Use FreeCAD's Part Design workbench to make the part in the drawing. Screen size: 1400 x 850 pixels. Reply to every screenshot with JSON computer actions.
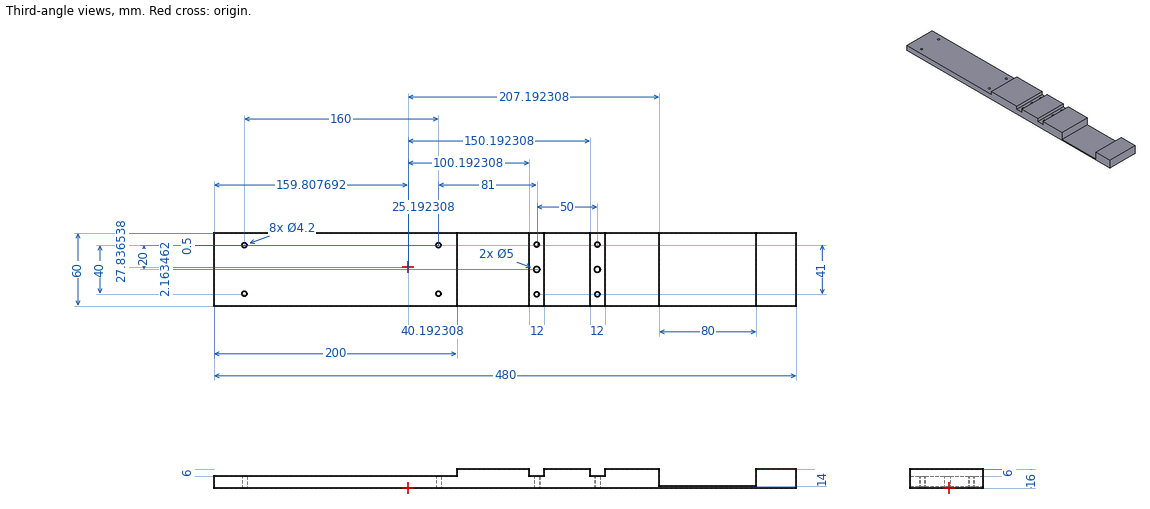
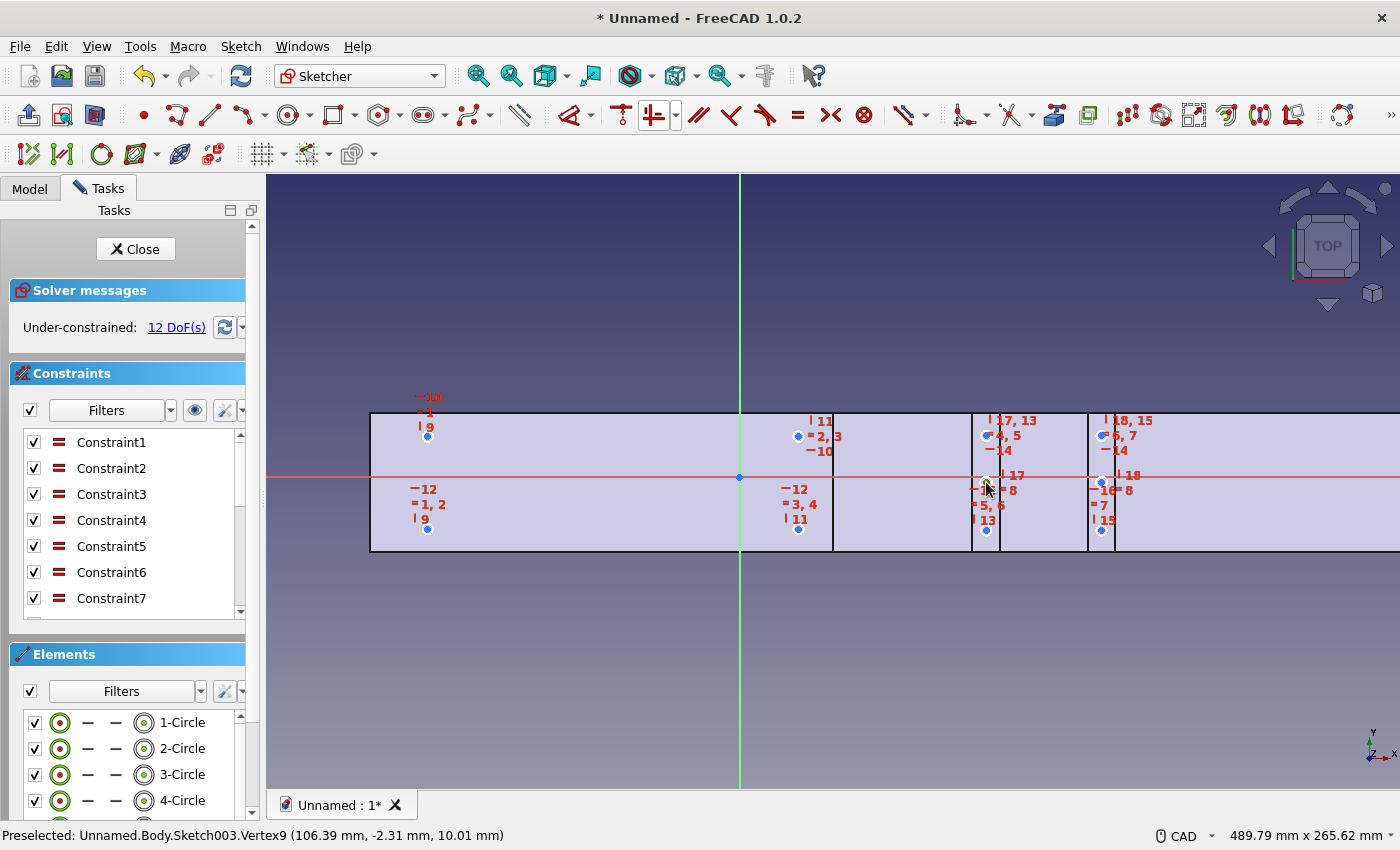
{"action": "left_click", "coordinate": [1102, 482]}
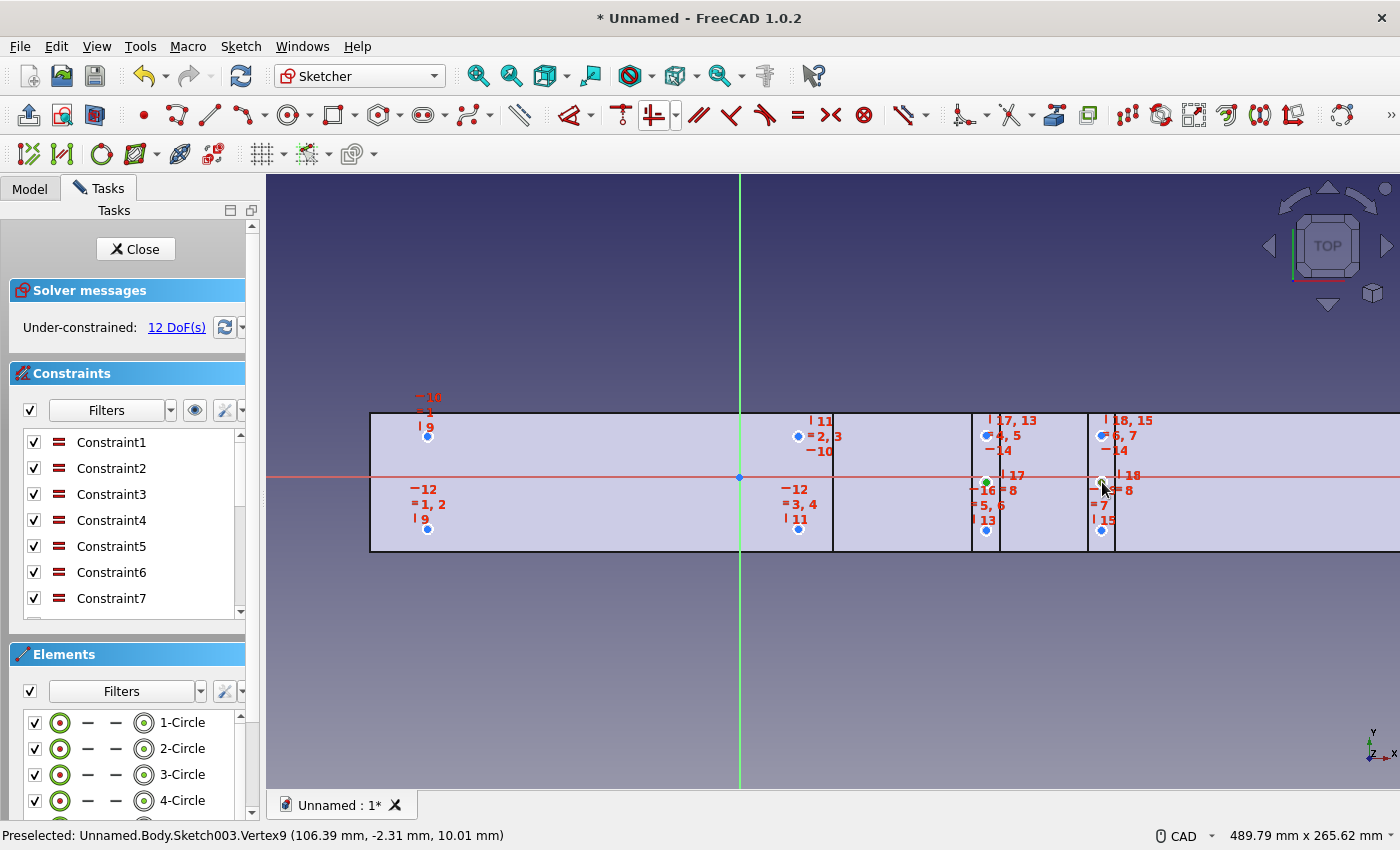
{"action": "key", "text": "h"}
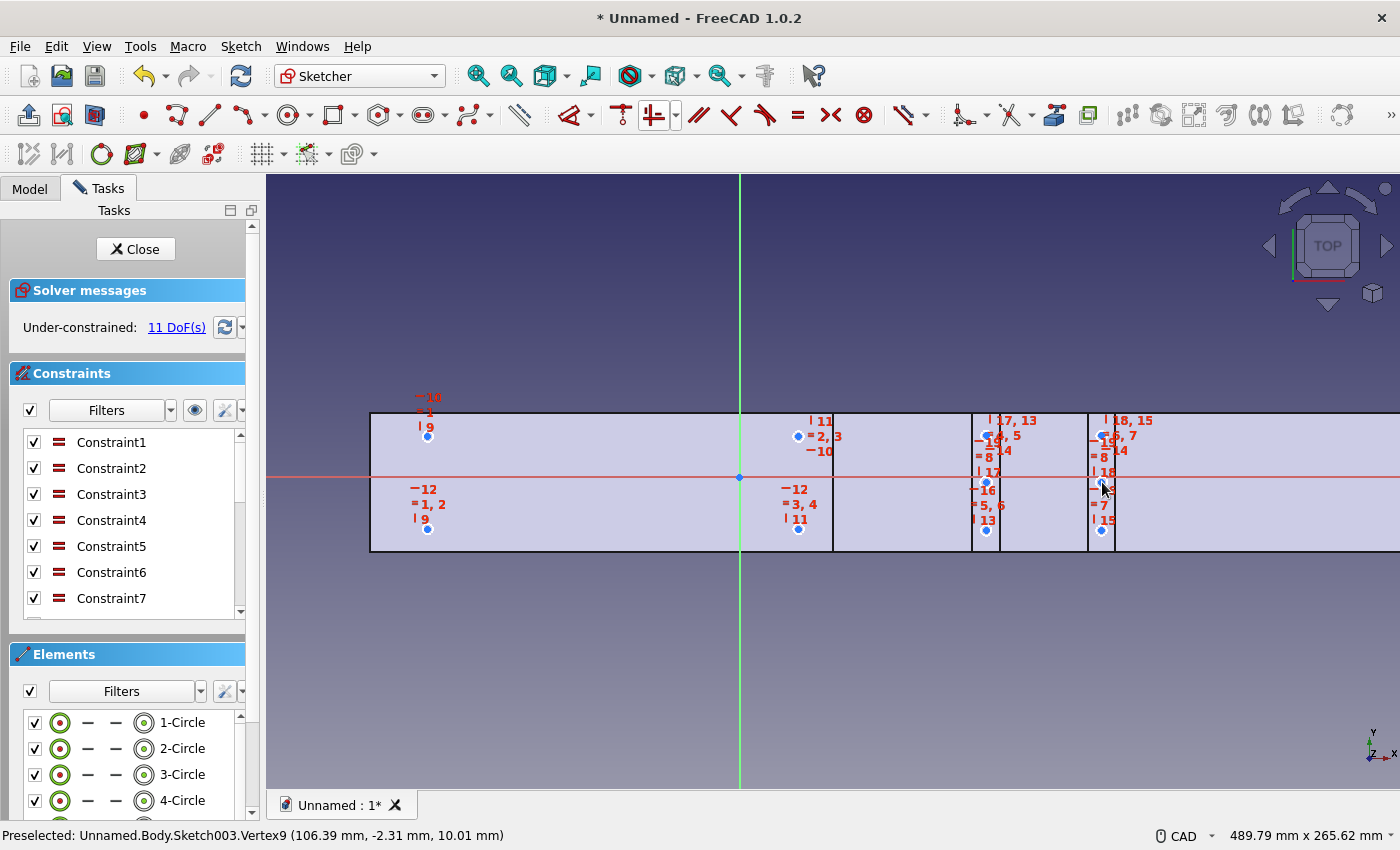
{"action": "key", "text": "d"}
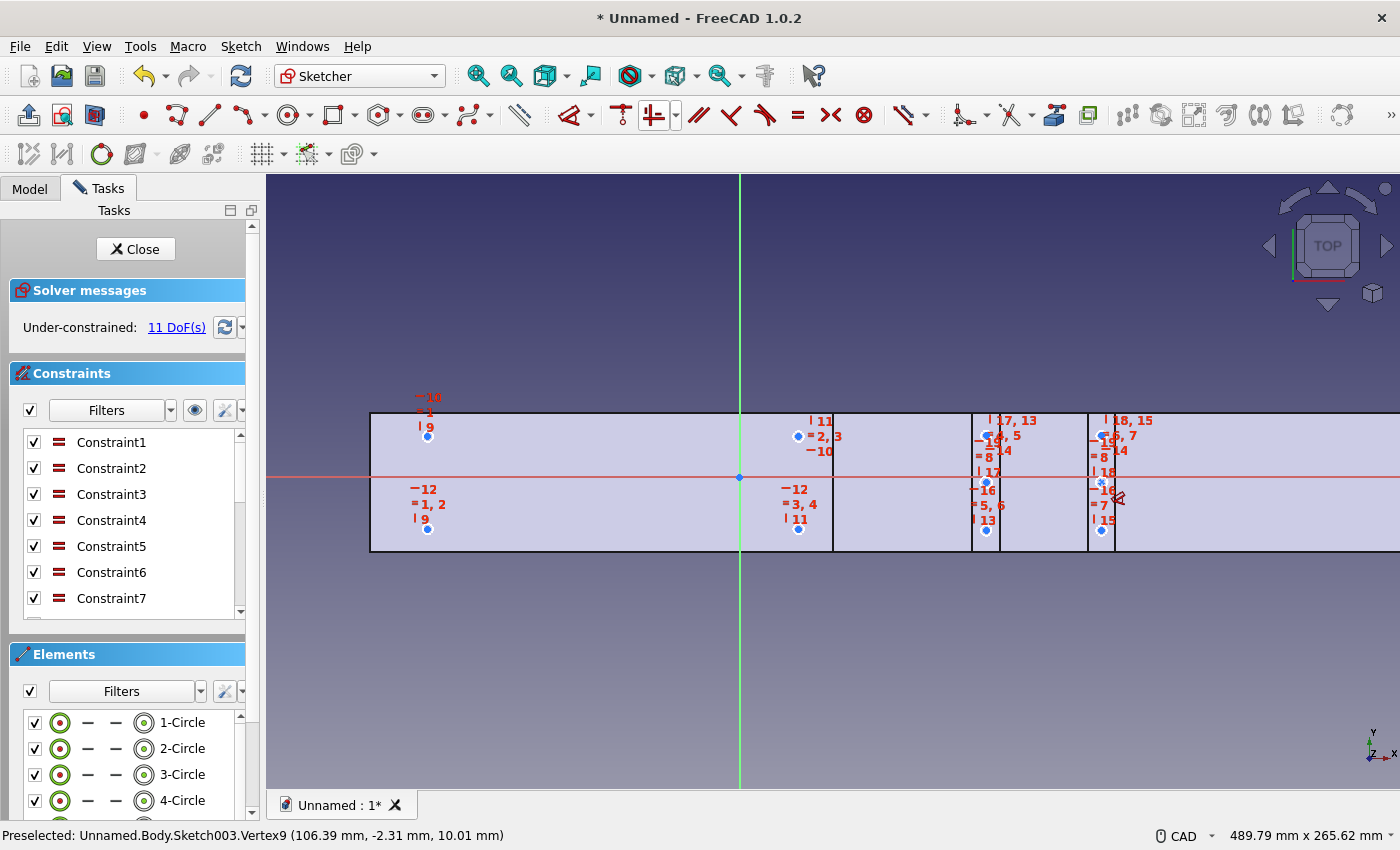
{"action": "scroll", "coordinate": [423, 436], "scroll_direction": "up", "scroll_amount": 8}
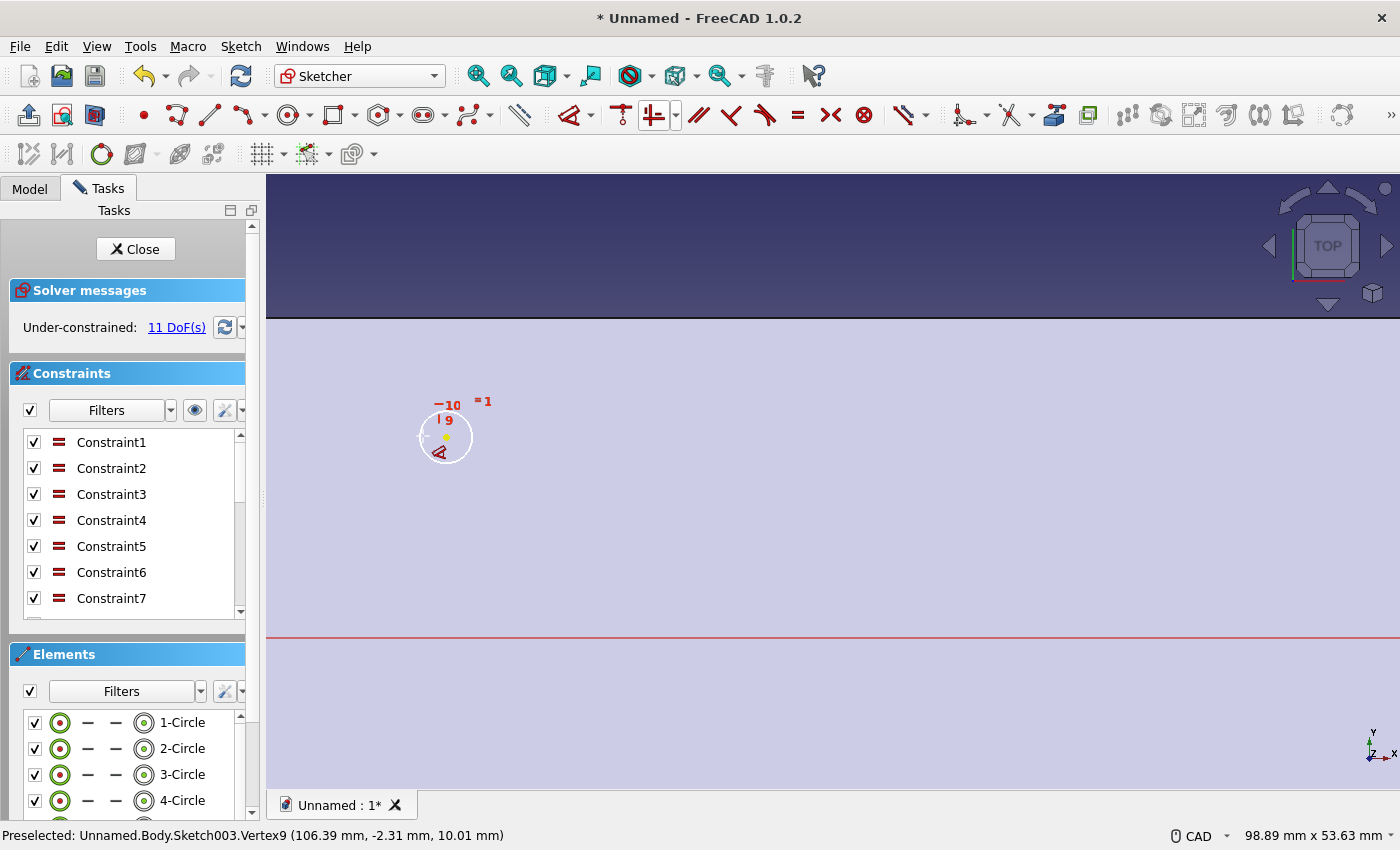
{"action": "left_click", "coordinate": [420, 437]}
{"action": "left_click", "coordinate": [388, 437]}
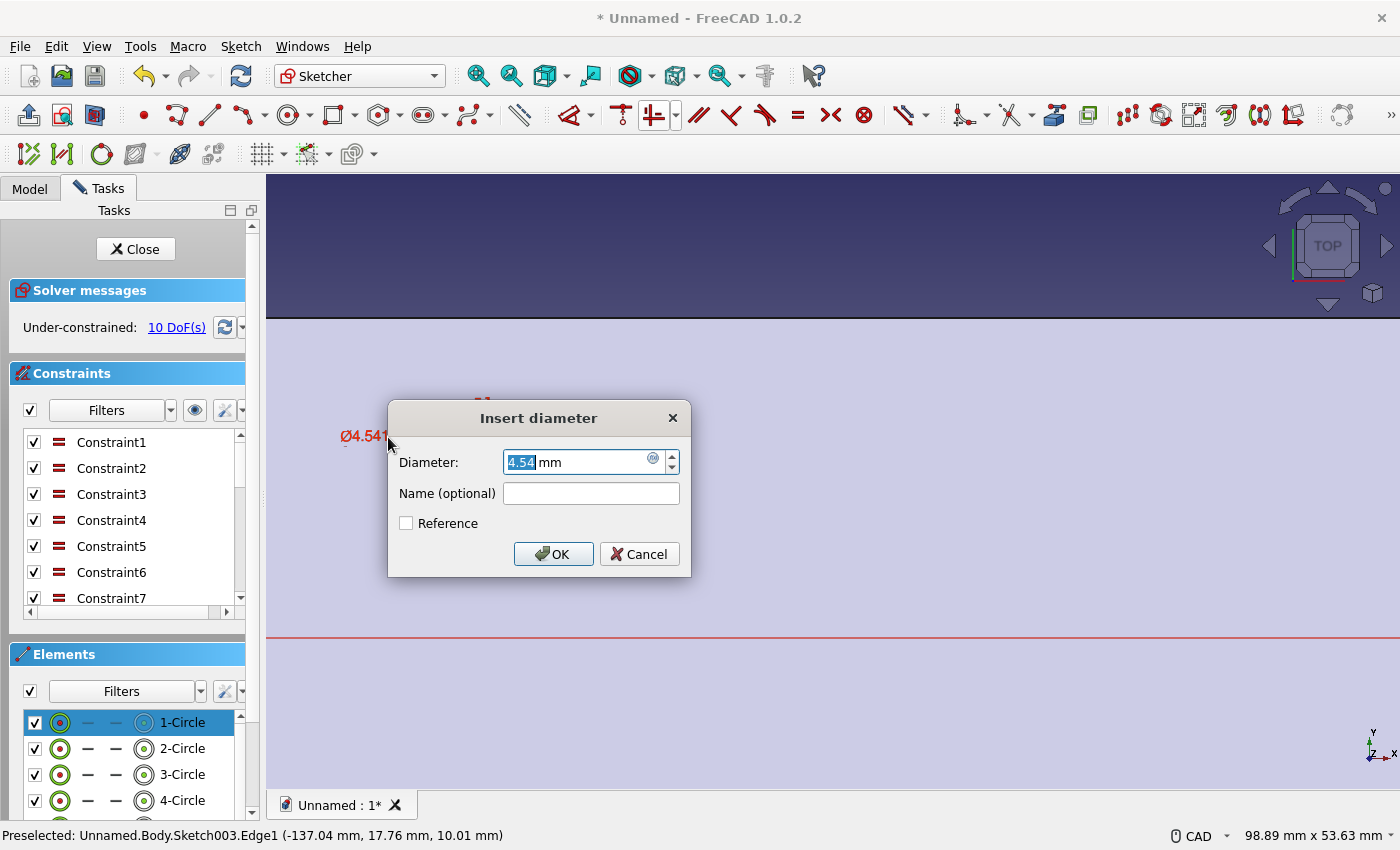
{"action": "type", "text": "4.2"}
{"action": "key", "text": "Return"}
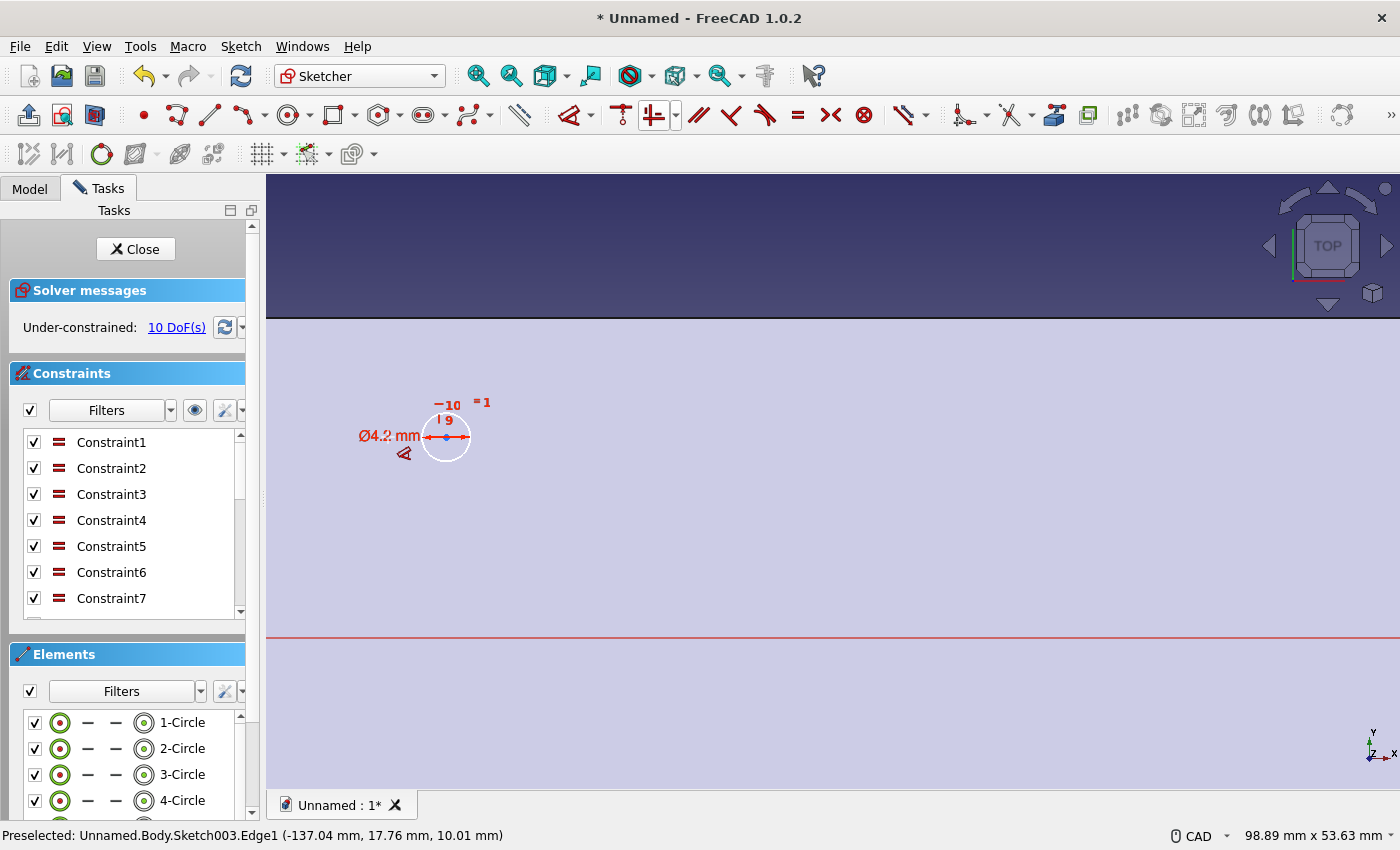
{"action": "scroll", "coordinate": [422, 436], "scroll_direction": "down", "scroll_amount": 8}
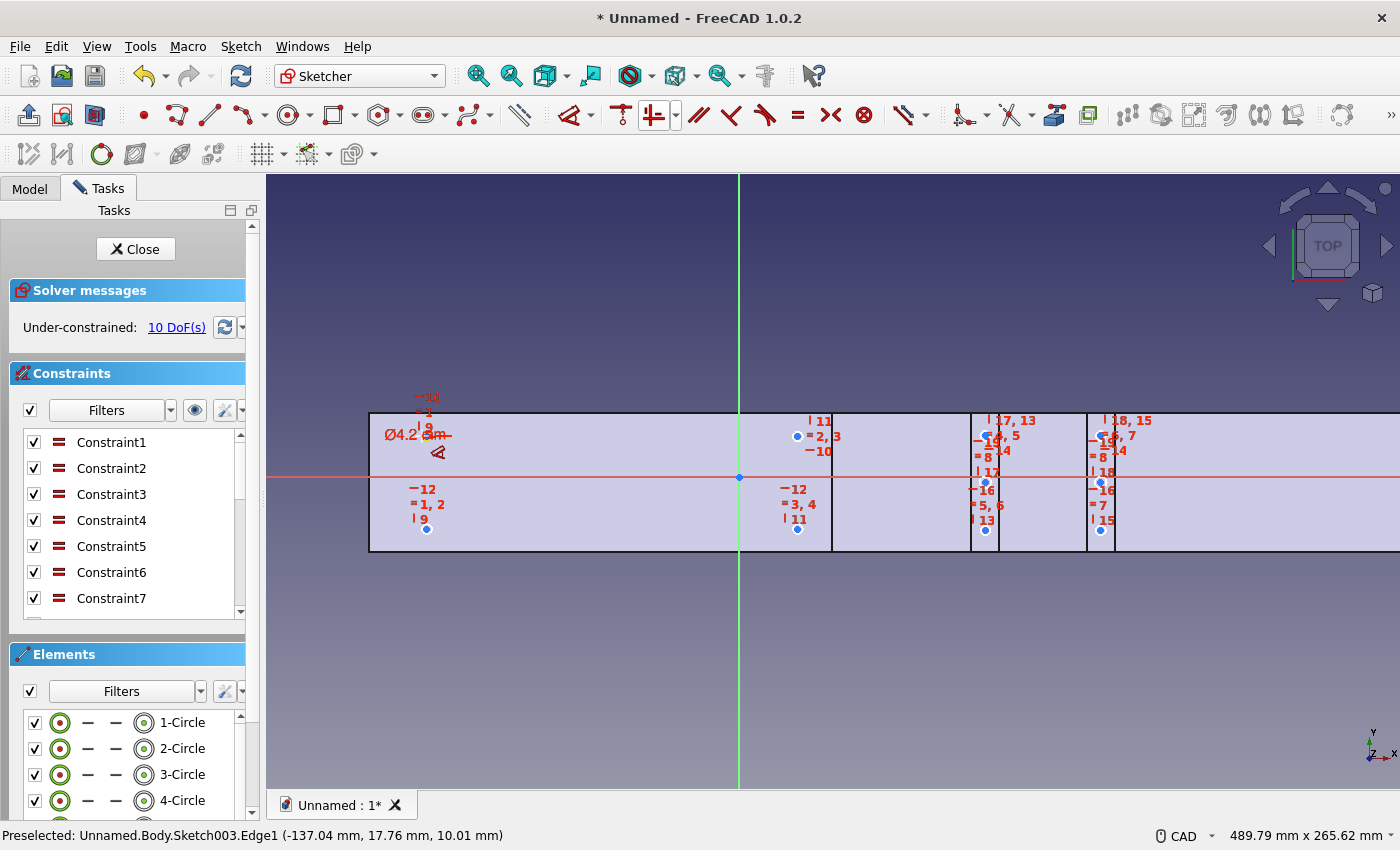
{"action": "scroll", "coordinate": [981, 487], "scroll_direction": "up", "scroll_amount": 7}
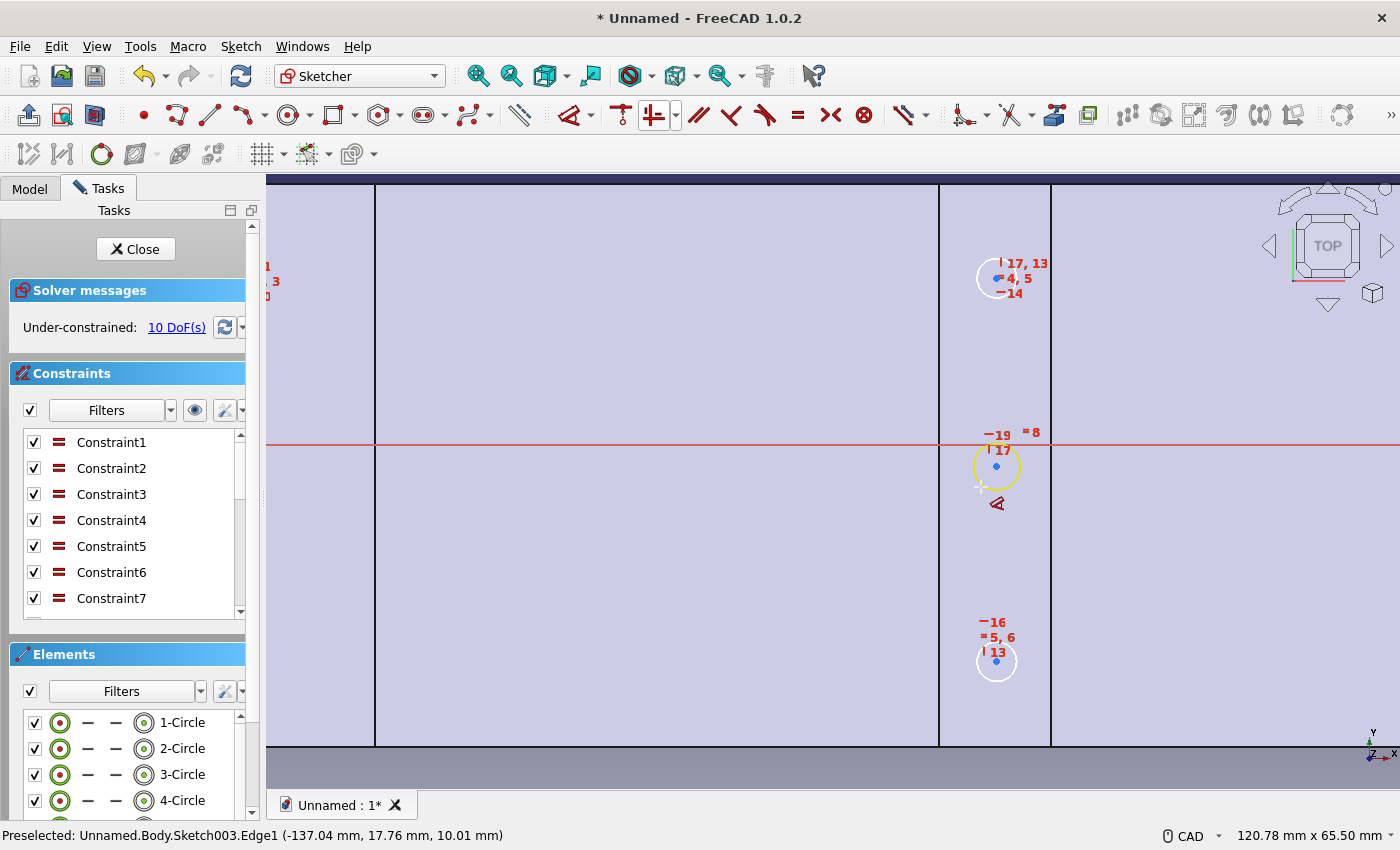
{"action": "left_click", "coordinate": [980, 483]}
{"action": "left_click", "coordinate": [957, 505]}